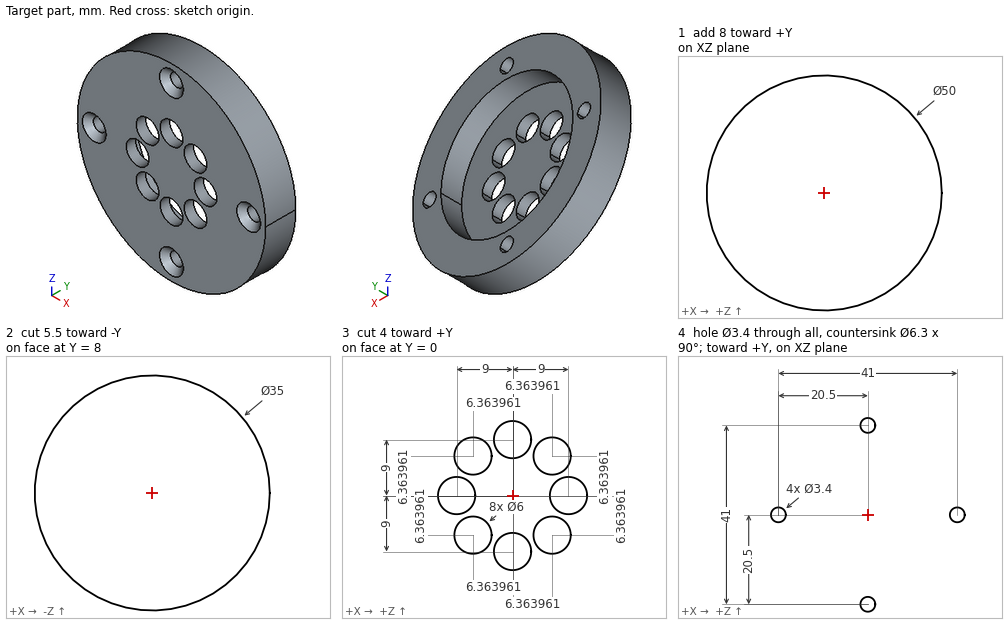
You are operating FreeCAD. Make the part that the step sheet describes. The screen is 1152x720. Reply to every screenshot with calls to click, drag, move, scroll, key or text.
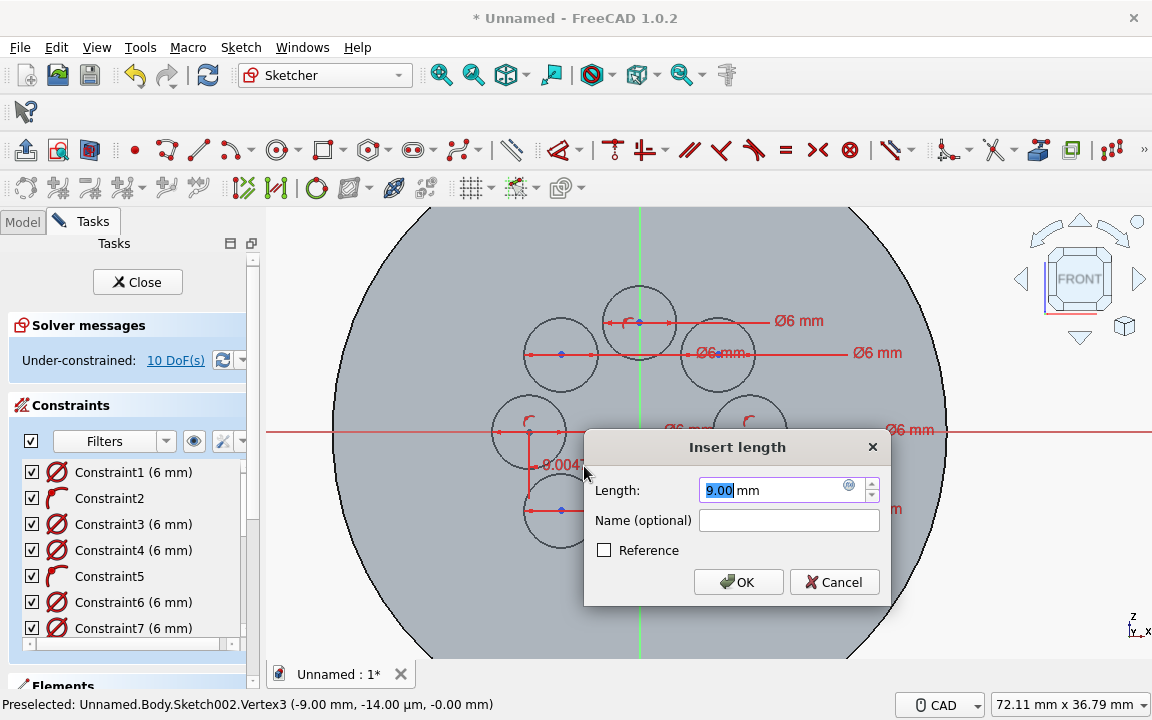
text(9)
key(Return)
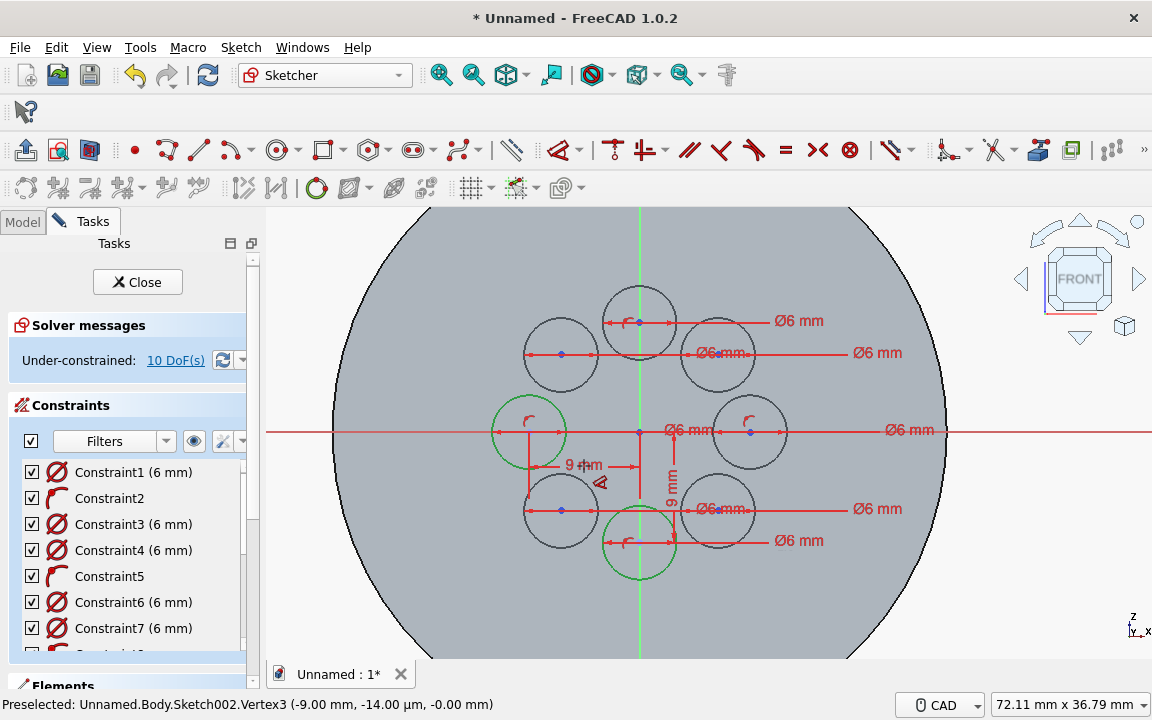
click(640, 323)
click(674, 403)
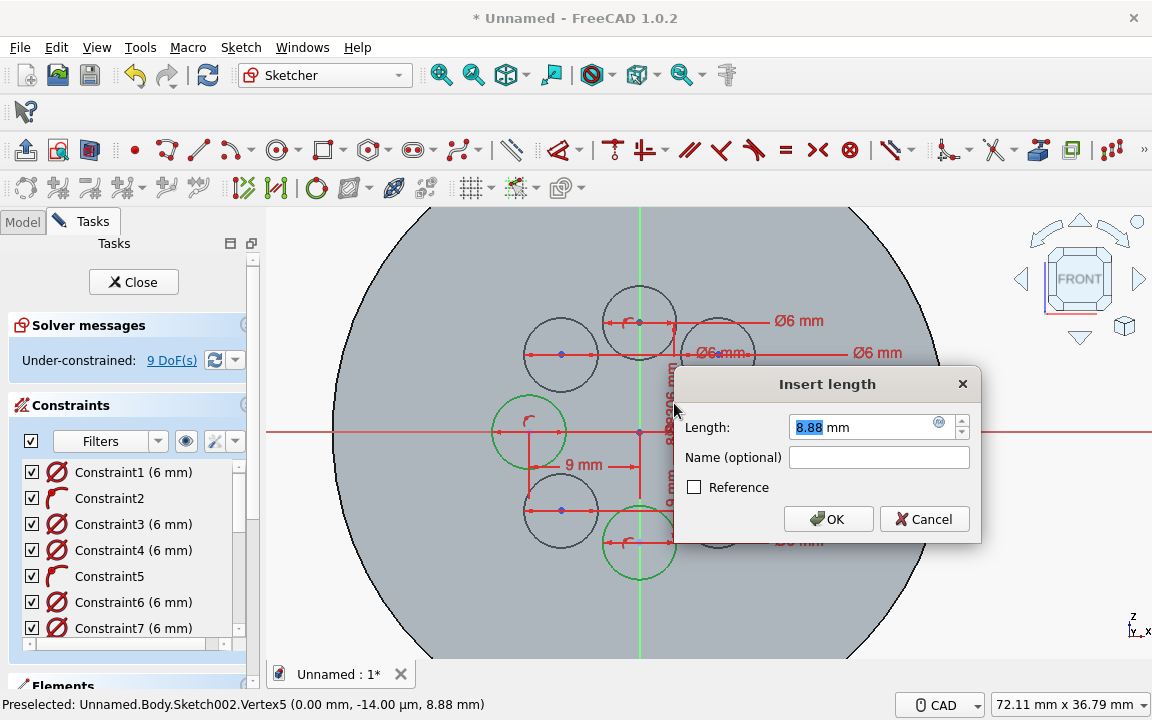
text(9)
key(Return)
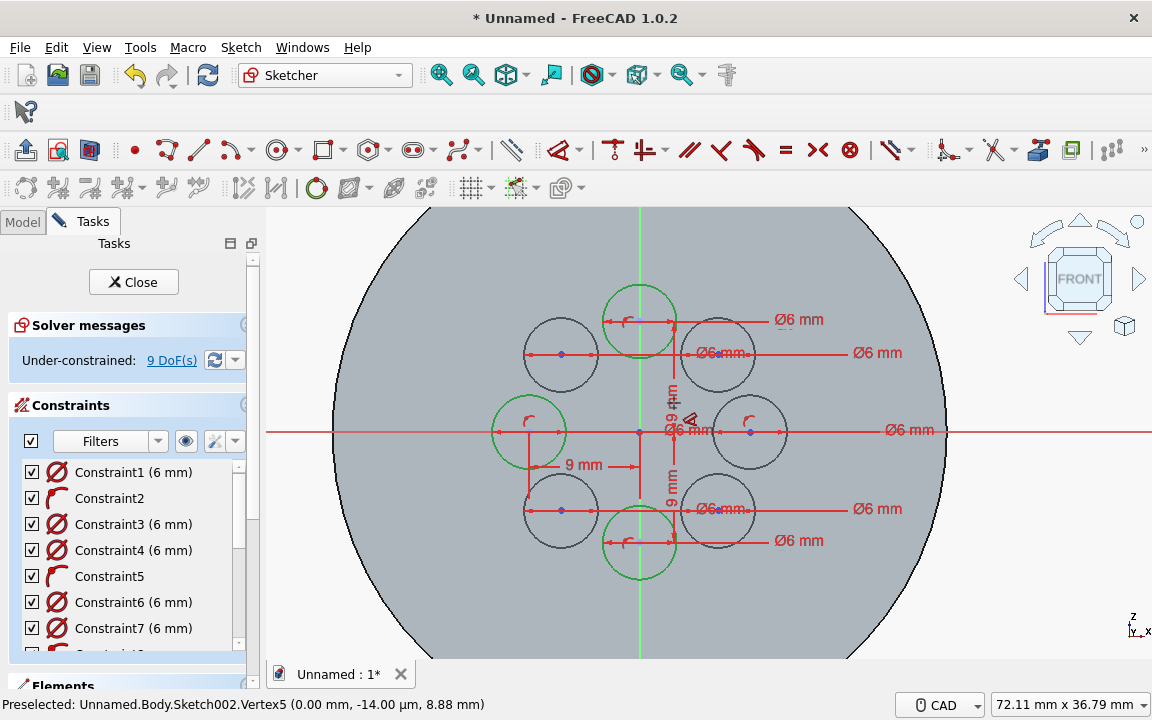
click(750, 432)
click(695, 466)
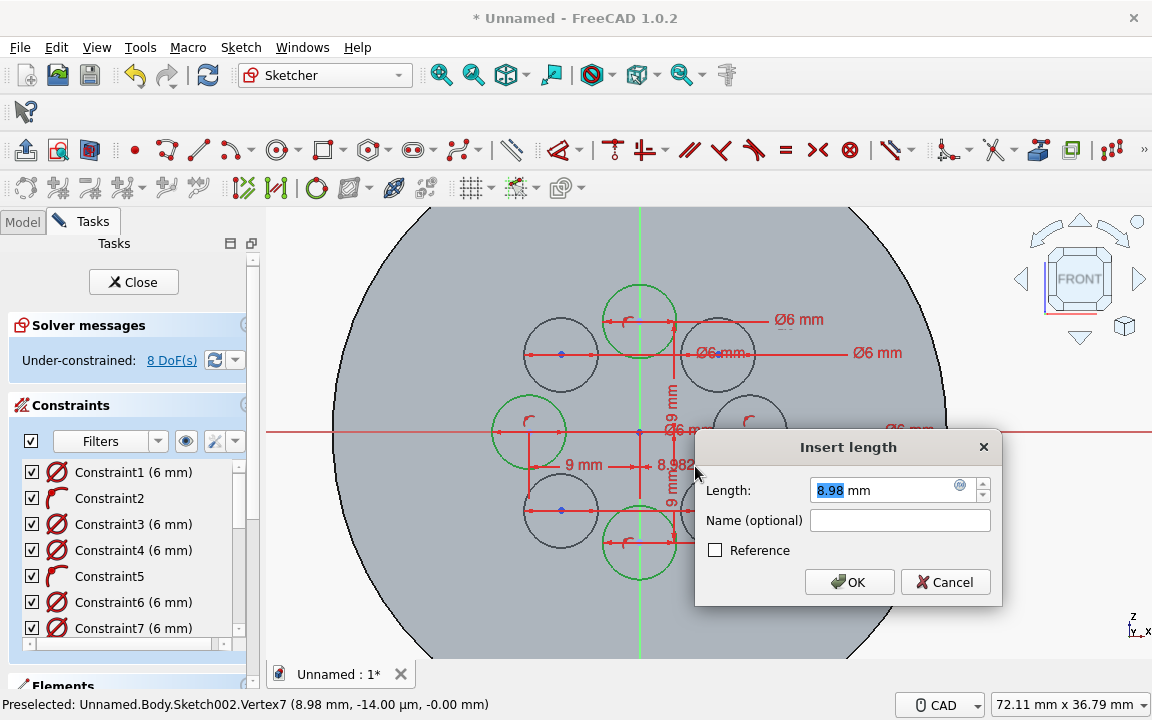
text(9)
key(Return)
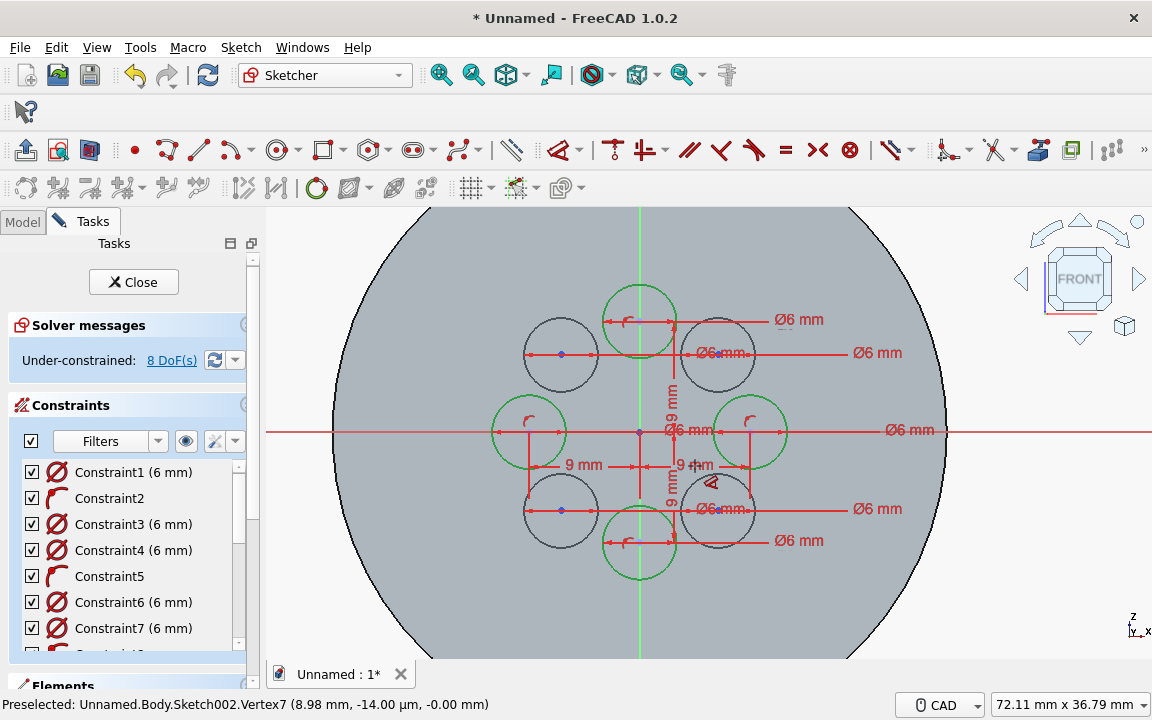
click(561, 511)
click(618, 545)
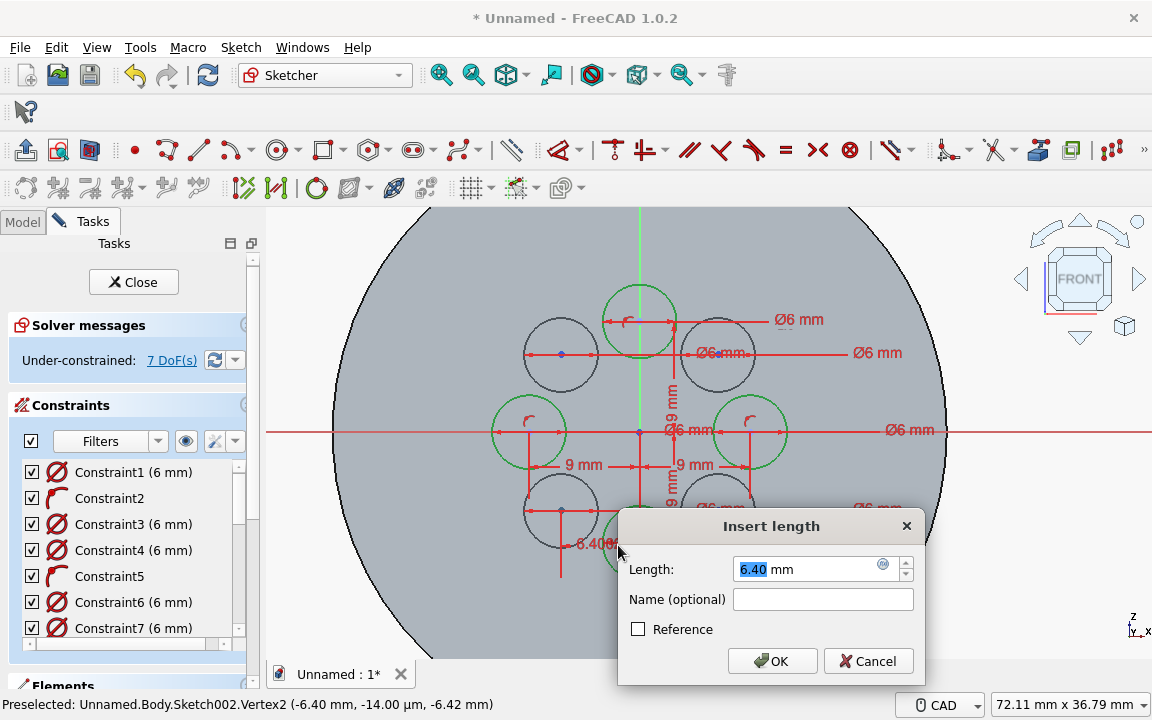
text(6.363961)
key(Return)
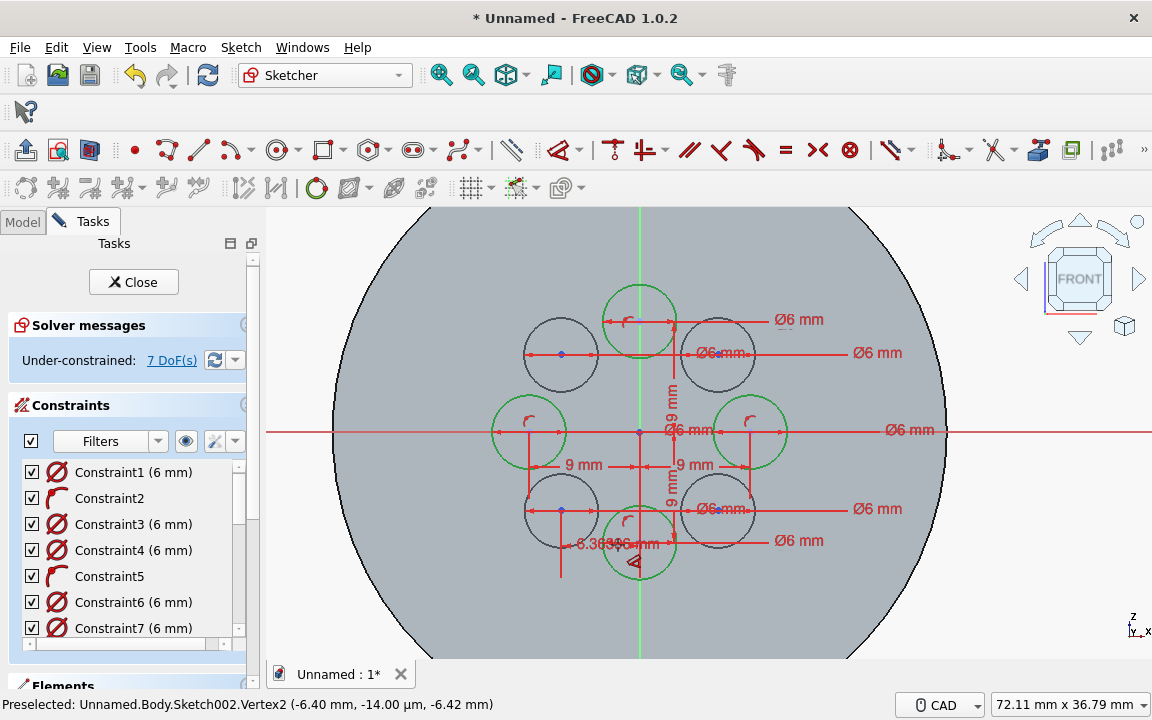
click(561, 511)
click(503, 490)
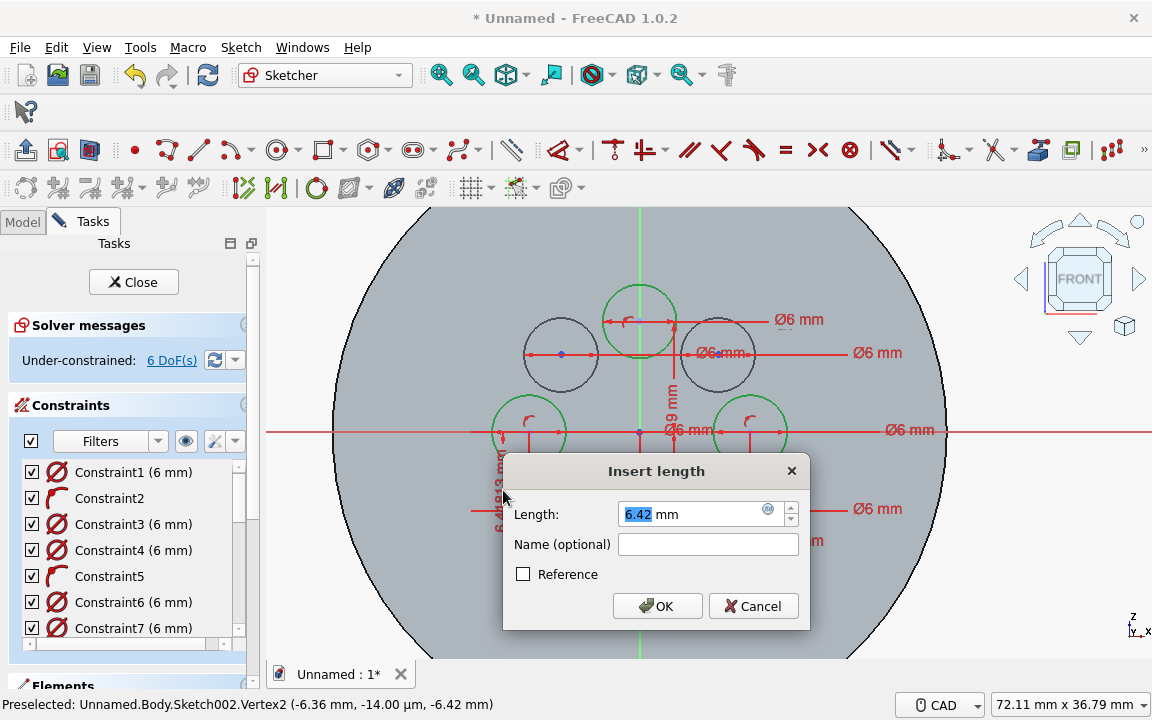
text(6.363961)
key(Return)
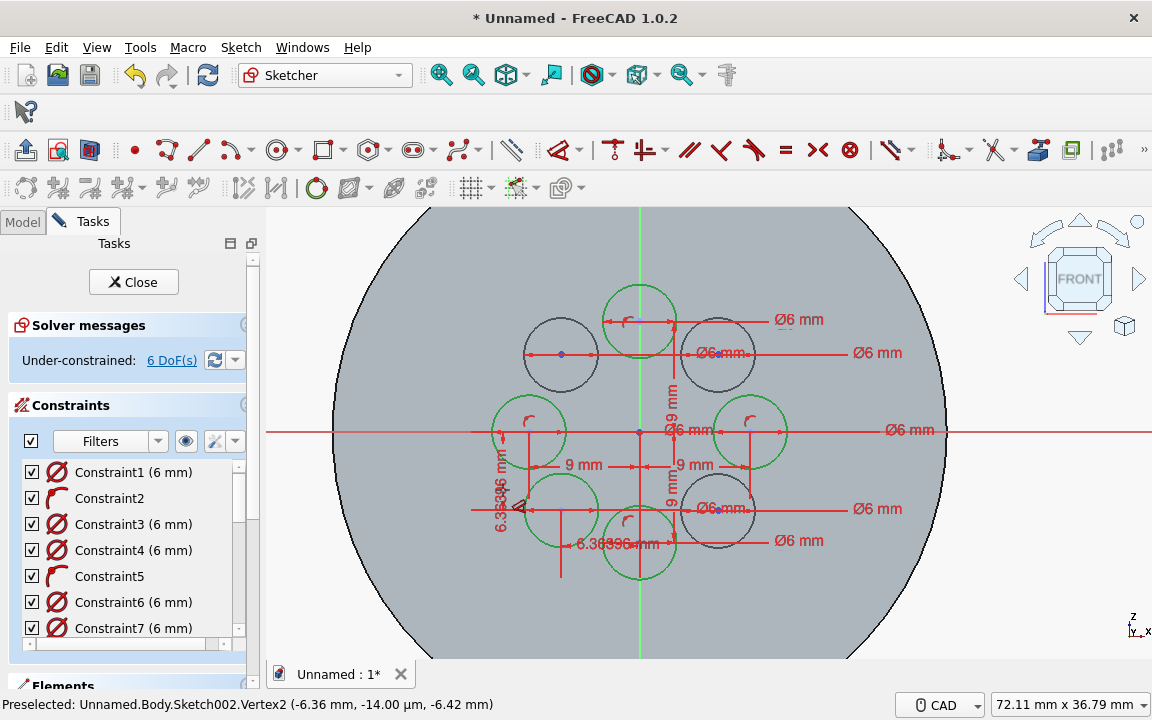
click(561, 355)
click(618, 321)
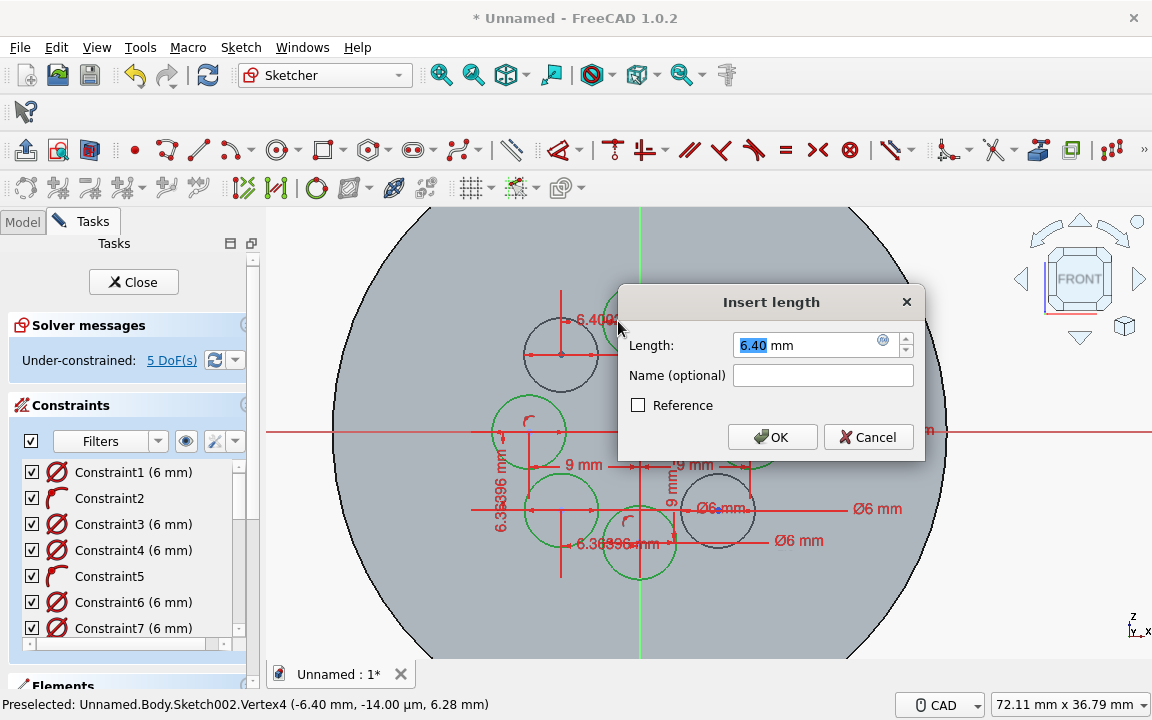
text(6.363961)
key(Return)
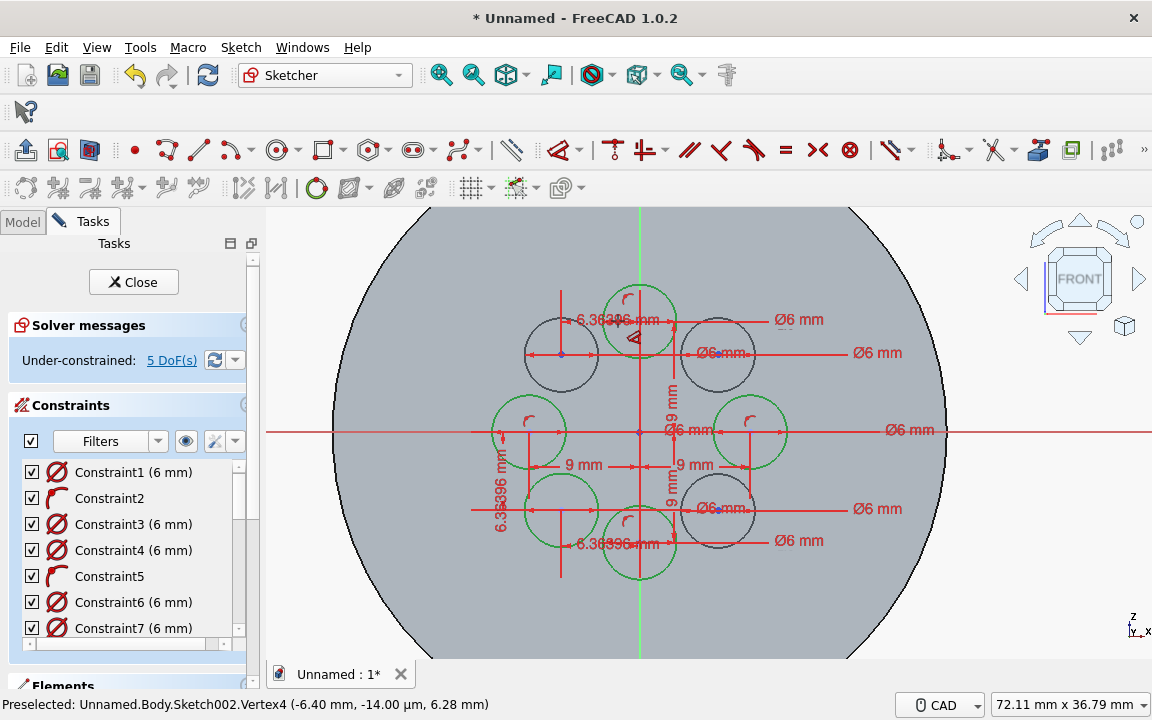
click(561, 355)
click(527, 411)